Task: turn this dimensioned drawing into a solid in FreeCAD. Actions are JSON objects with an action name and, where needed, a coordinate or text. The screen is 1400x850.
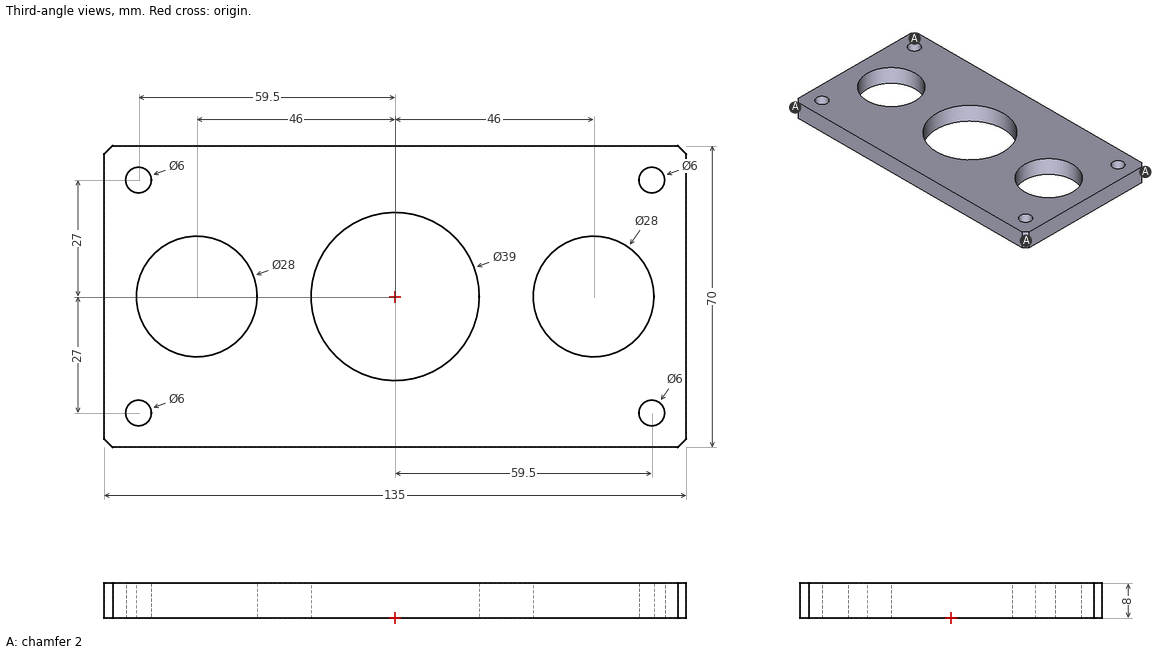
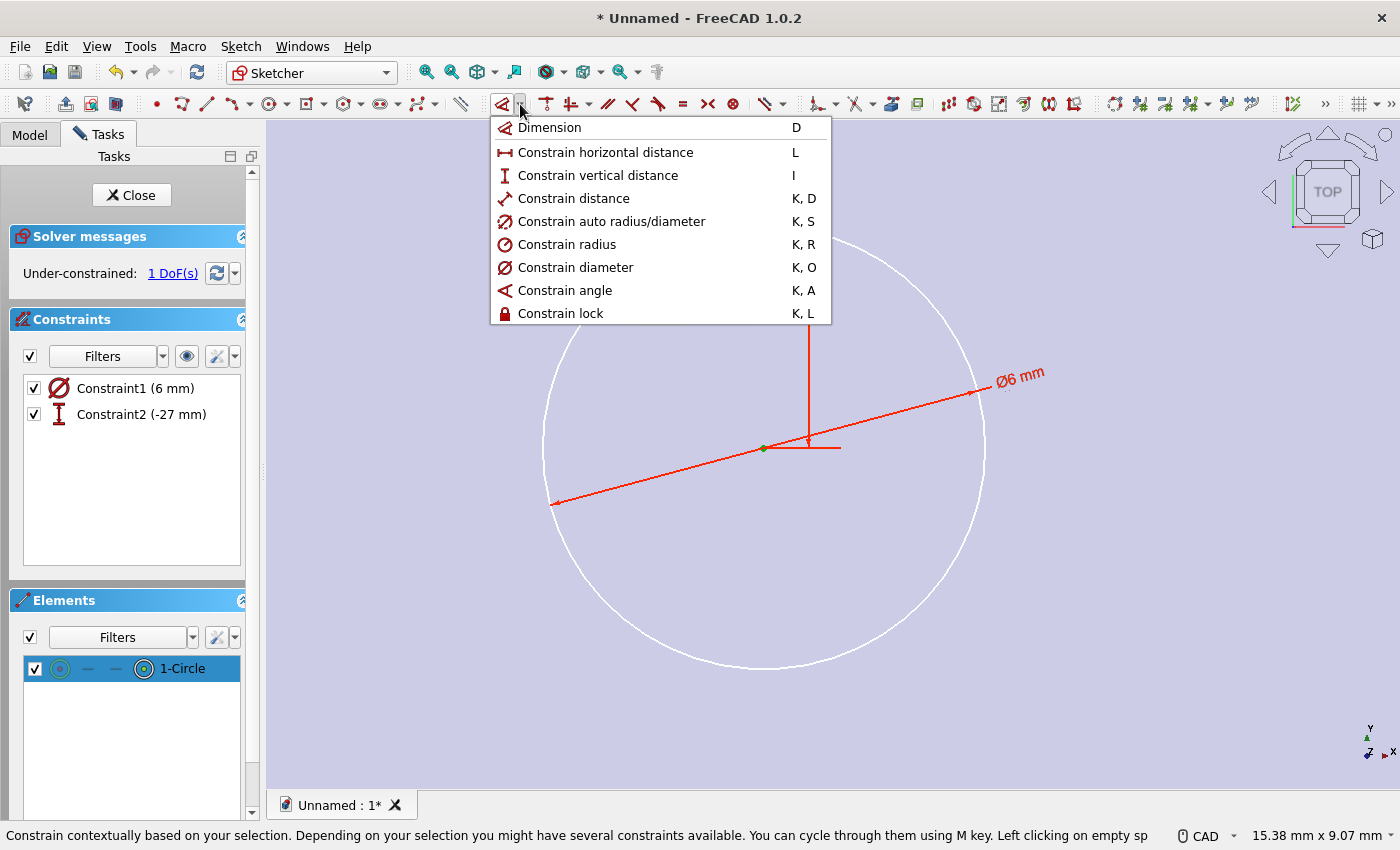
{"action": "left_click", "coordinate": [661, 152]}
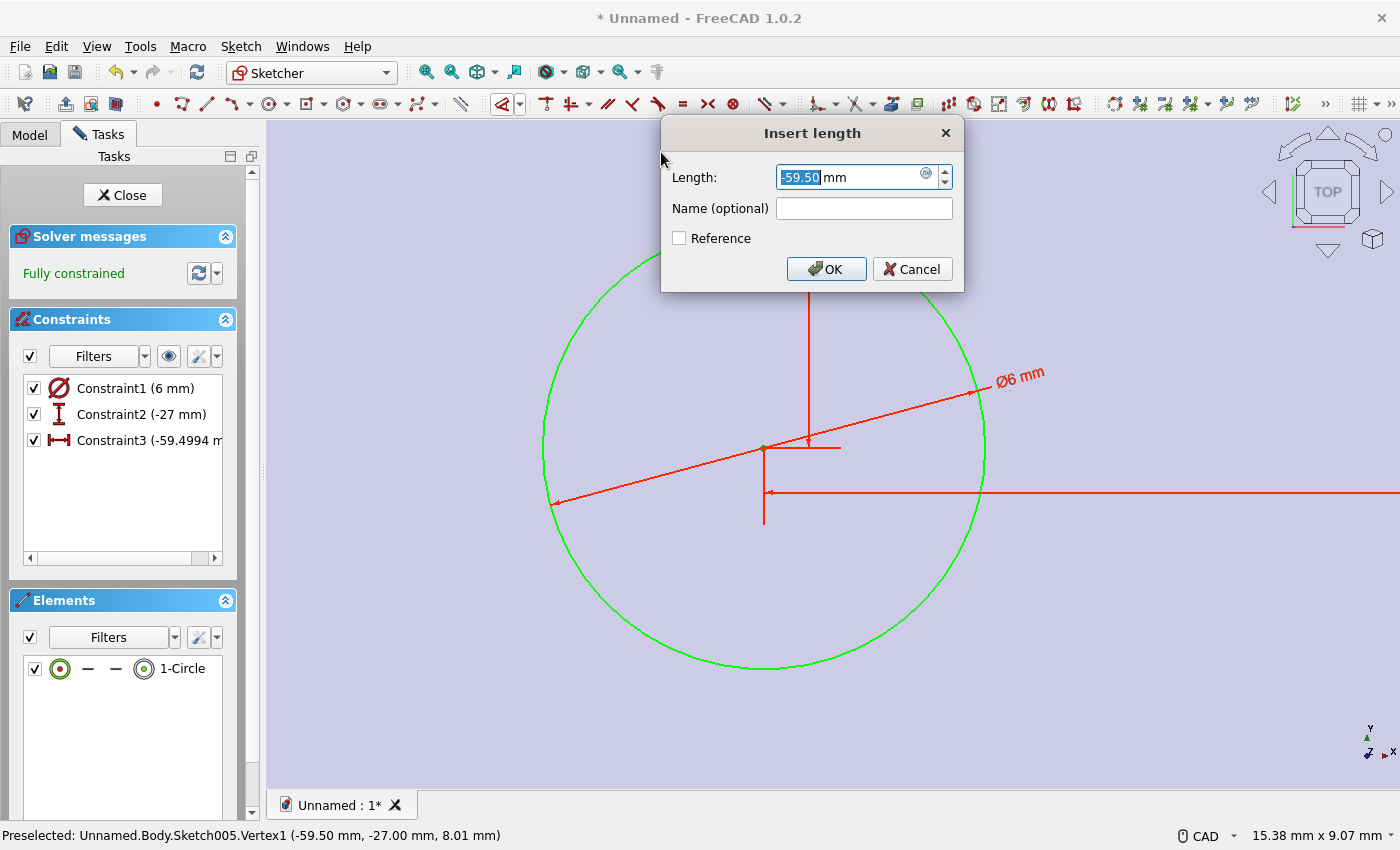
{"action": "type", "text": "-59.5"}
{"action": "key", "text": "Return"}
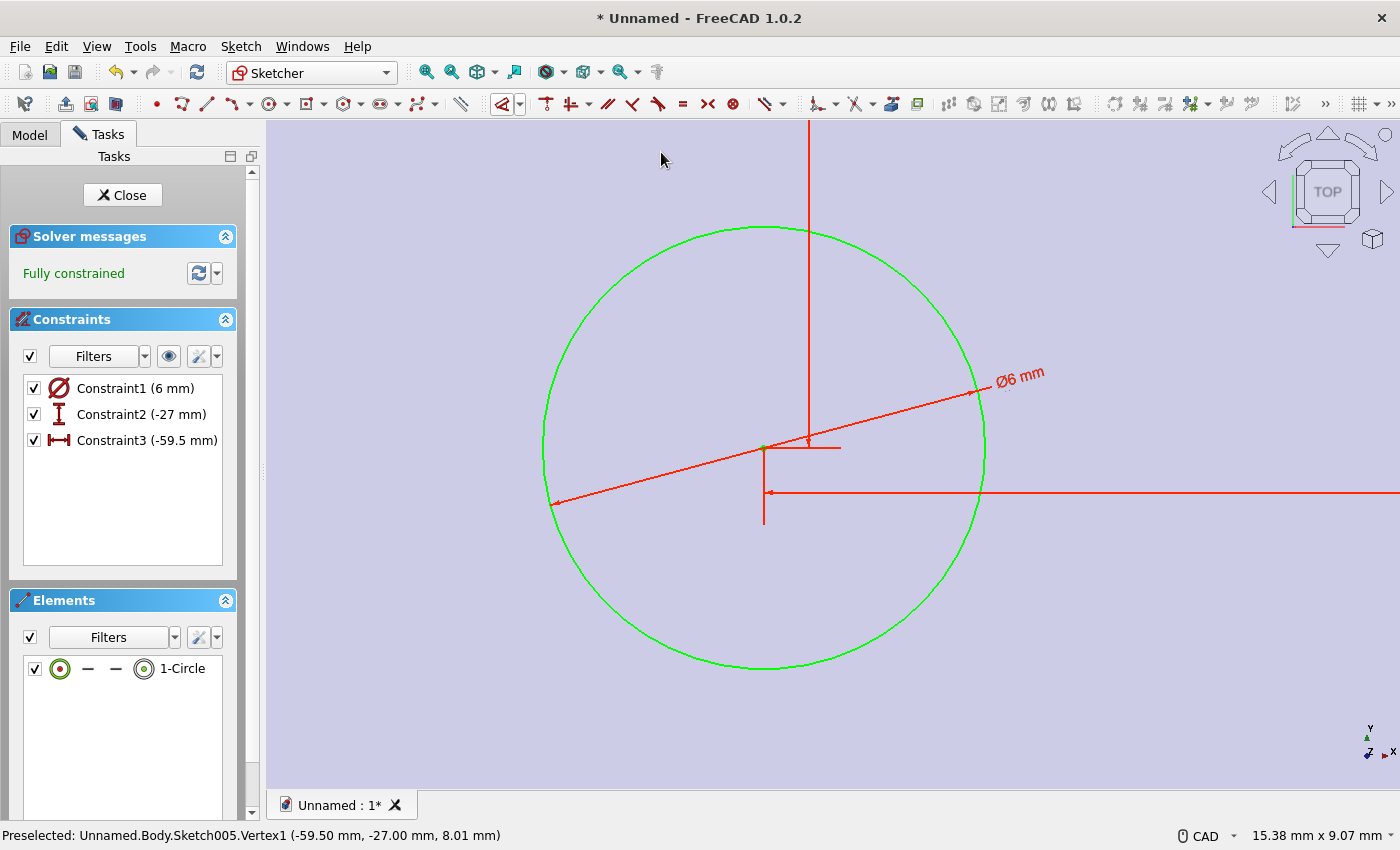
{"action": "left_click", "coordinate": [123, 195]}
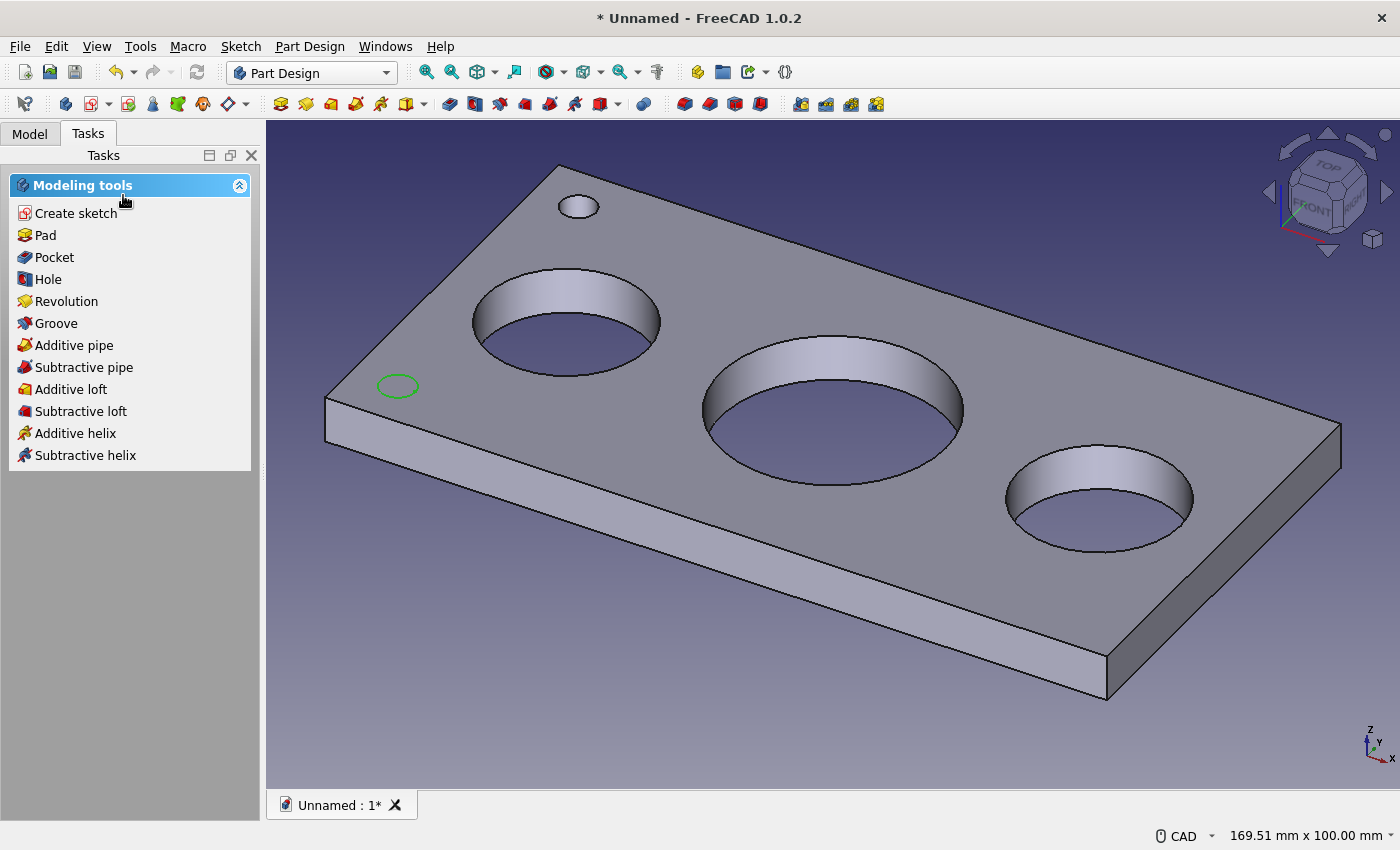
{"action": "left_click", "coordinate": [450, 104]}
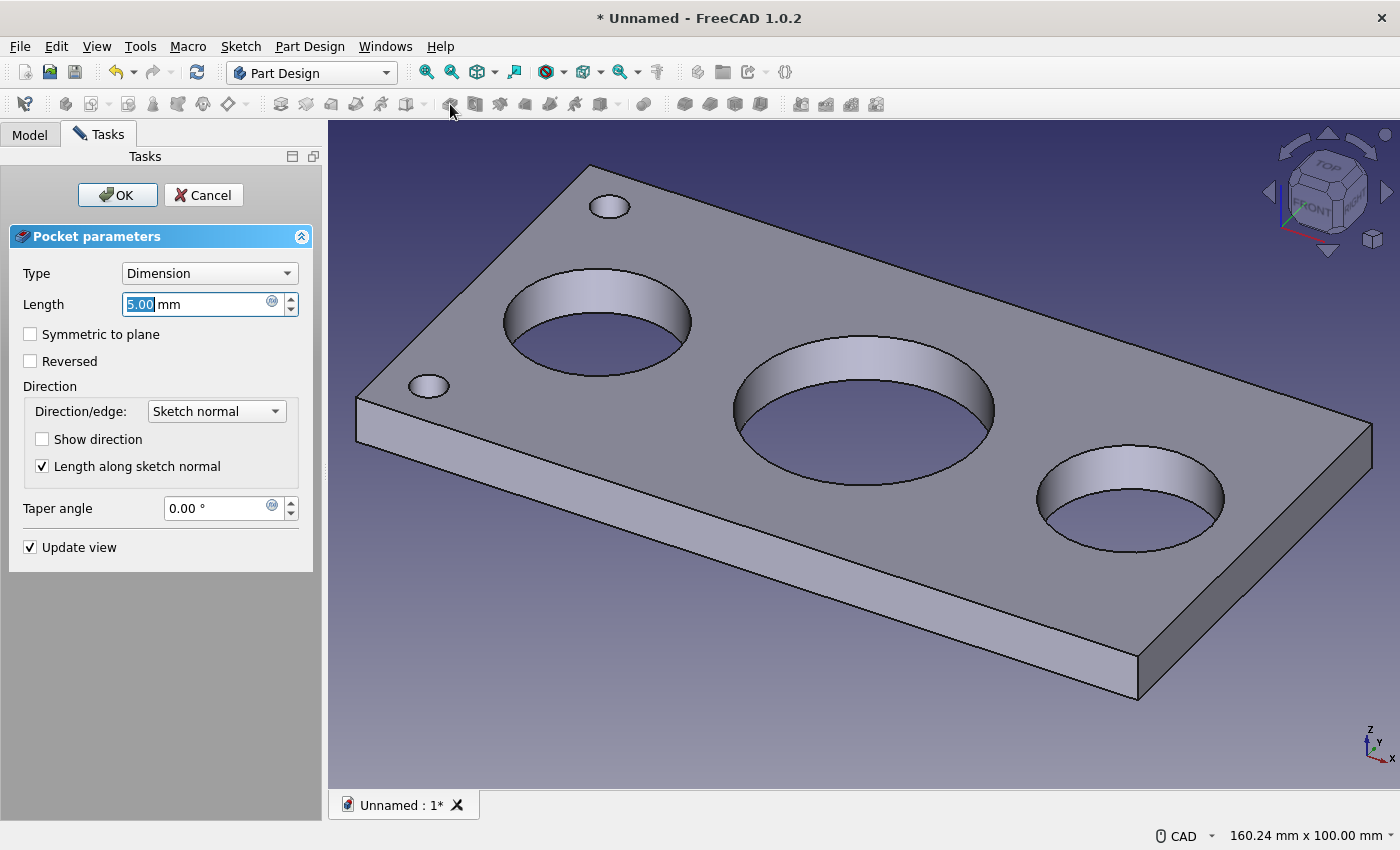
{"action": "left_click", "coordinate": [210, 274]}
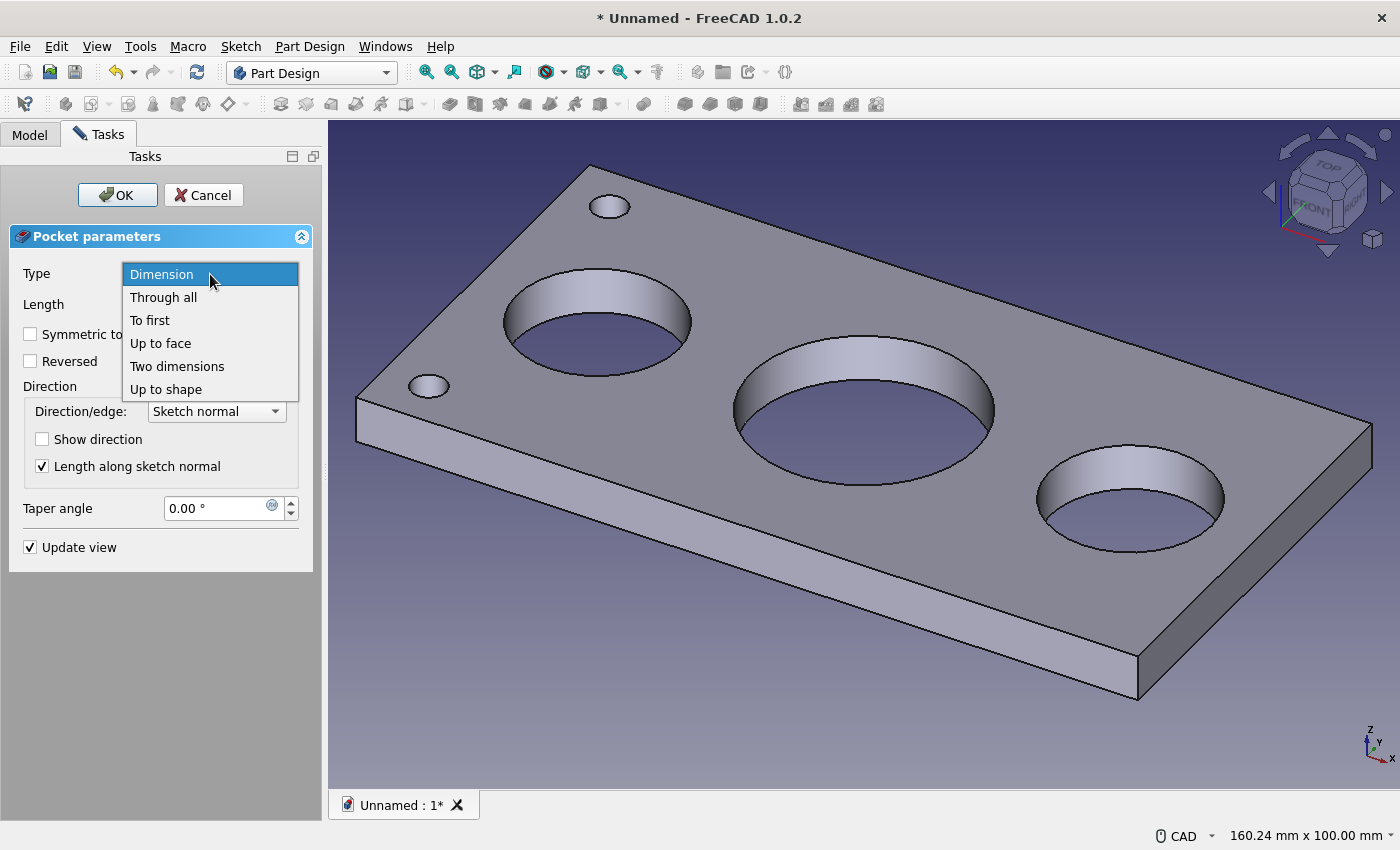
{"action": "left_click", "coordinate": [208, 320]}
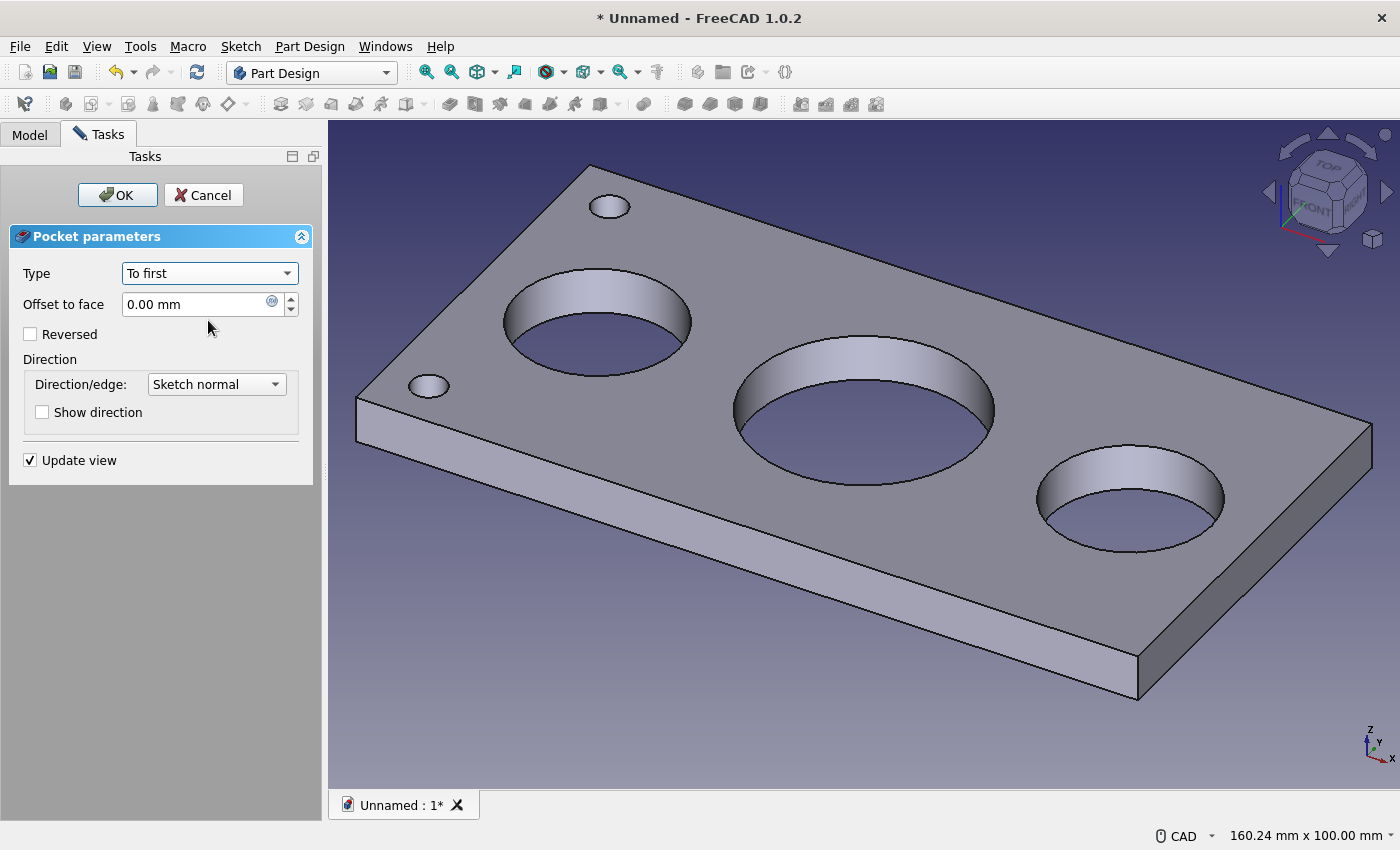
{"action": "left_click", "coordinate": [118, 195]}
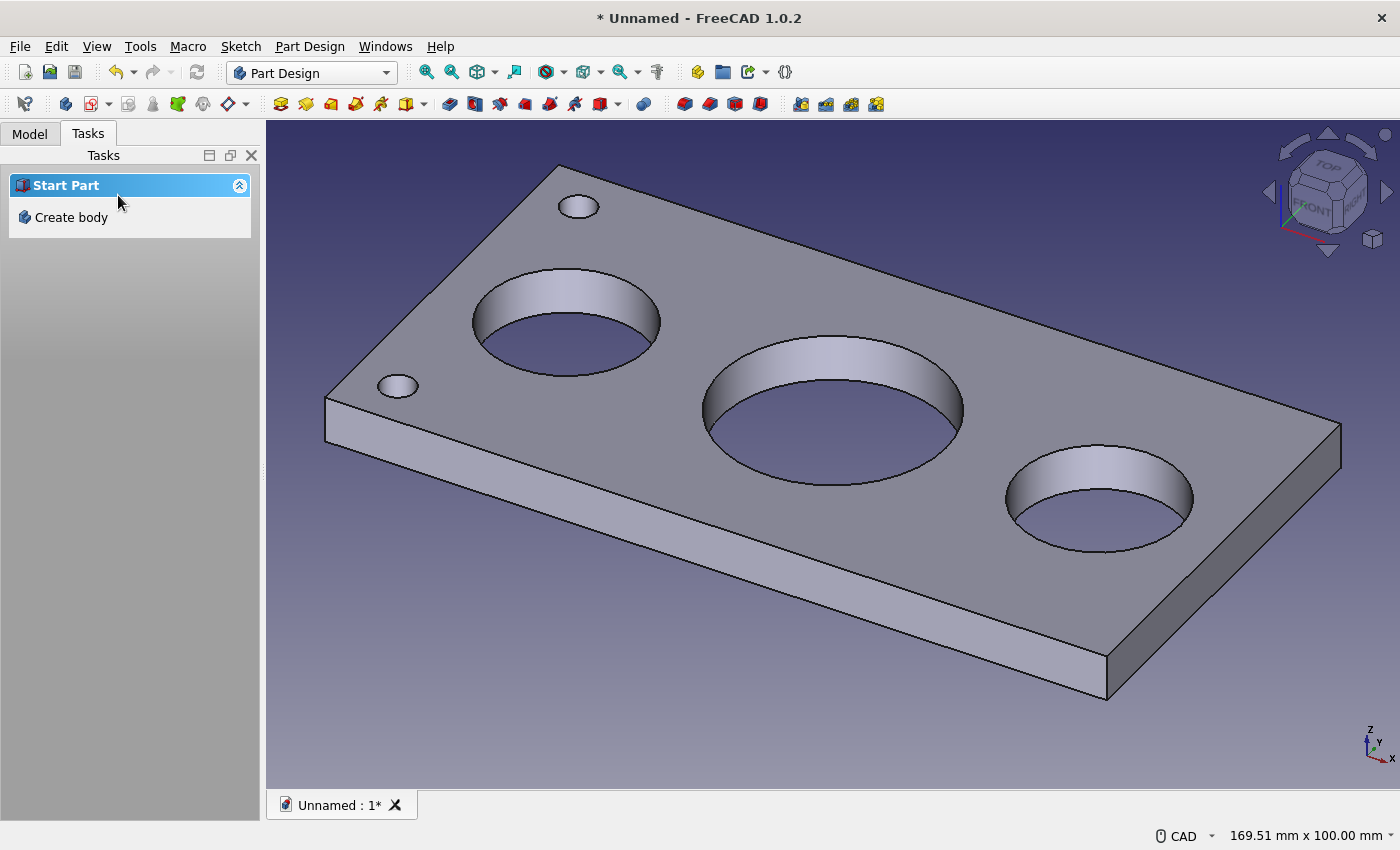
{"action": "left_click", "coordinate": [1235, 454]}